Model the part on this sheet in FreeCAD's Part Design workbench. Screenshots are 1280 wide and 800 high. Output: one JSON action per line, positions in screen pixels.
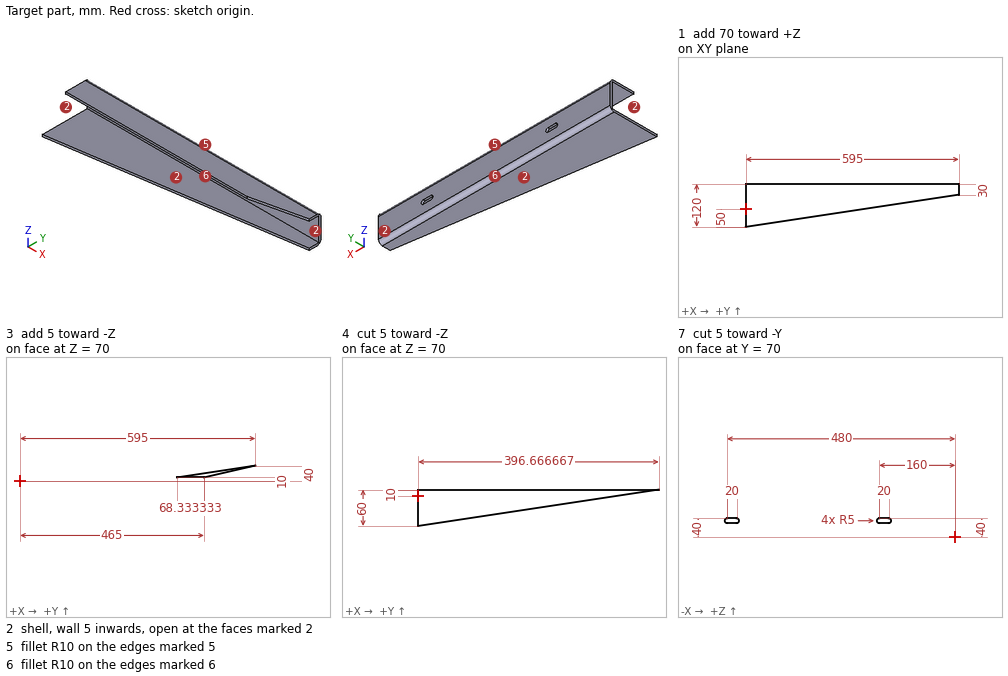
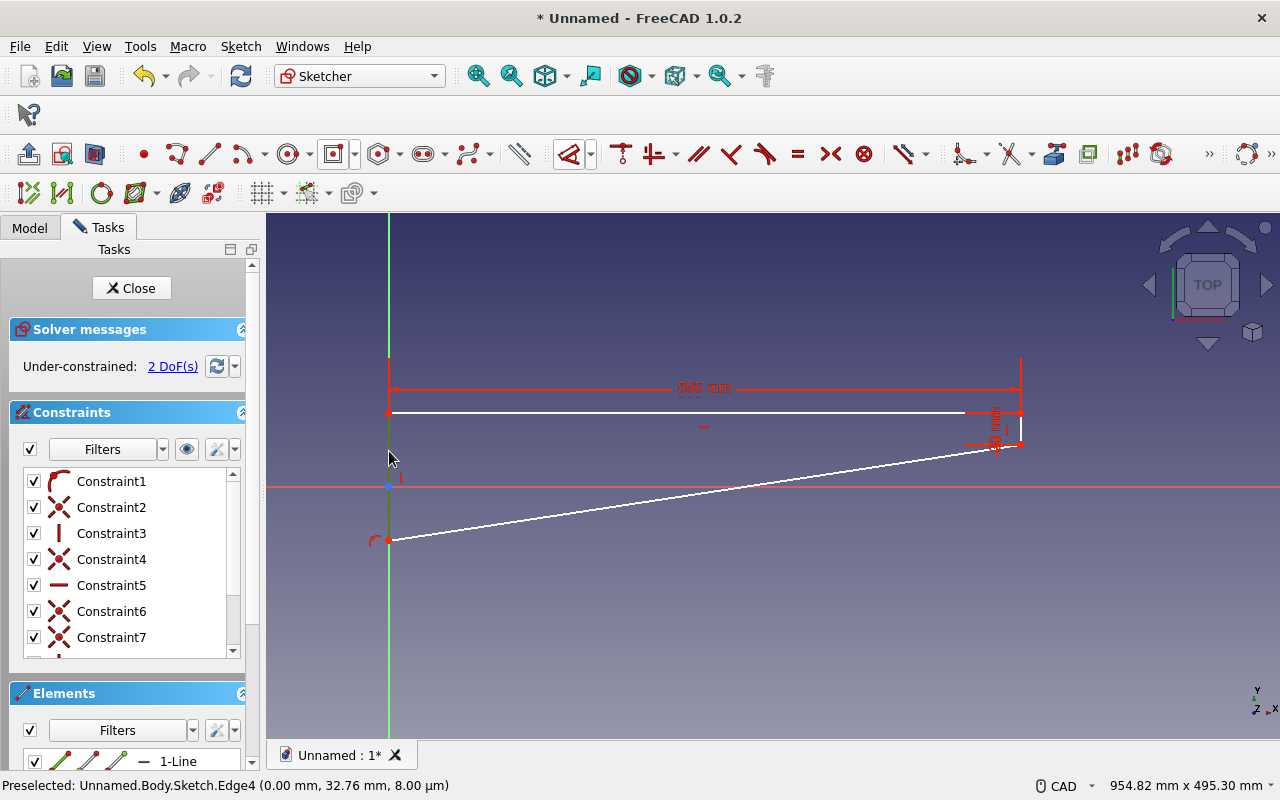
{"action": "left_click", "coordinate": [590, 154]}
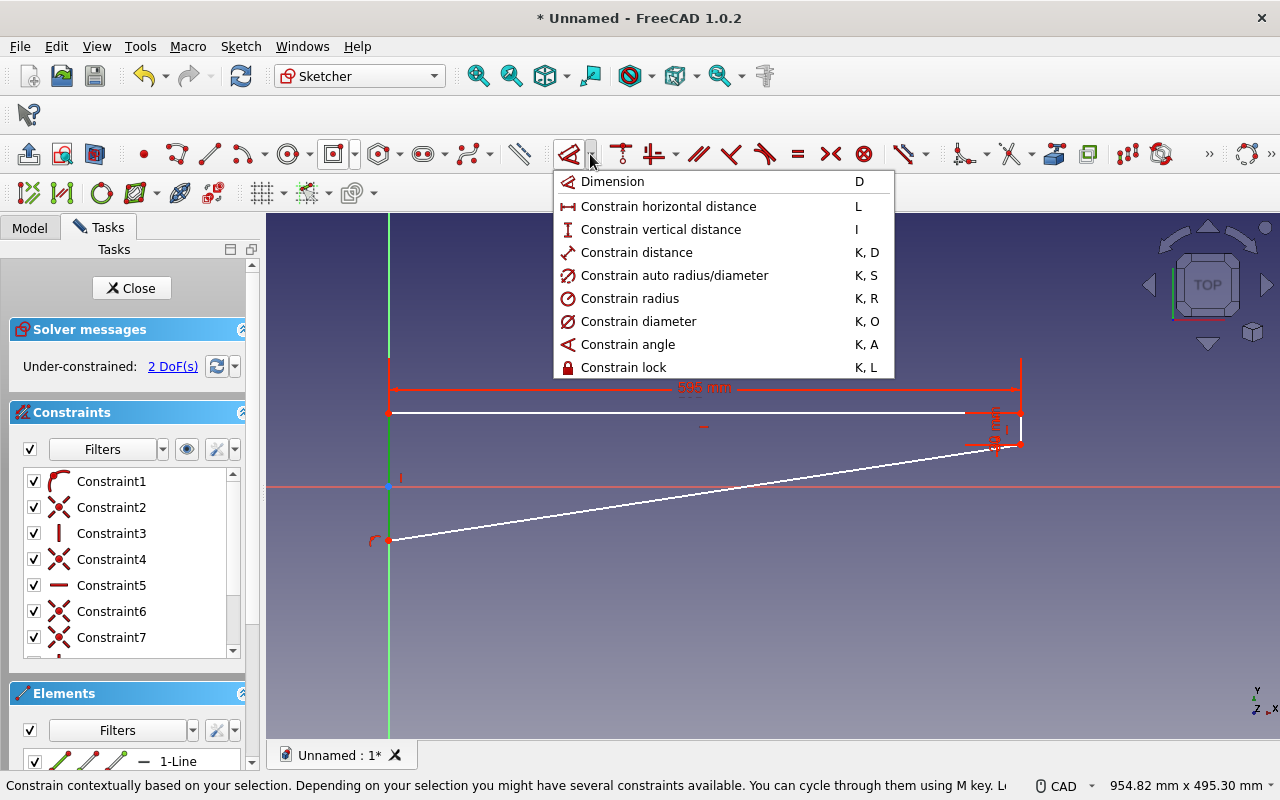
{"action": "left_click", "coordinate": [724, 230]}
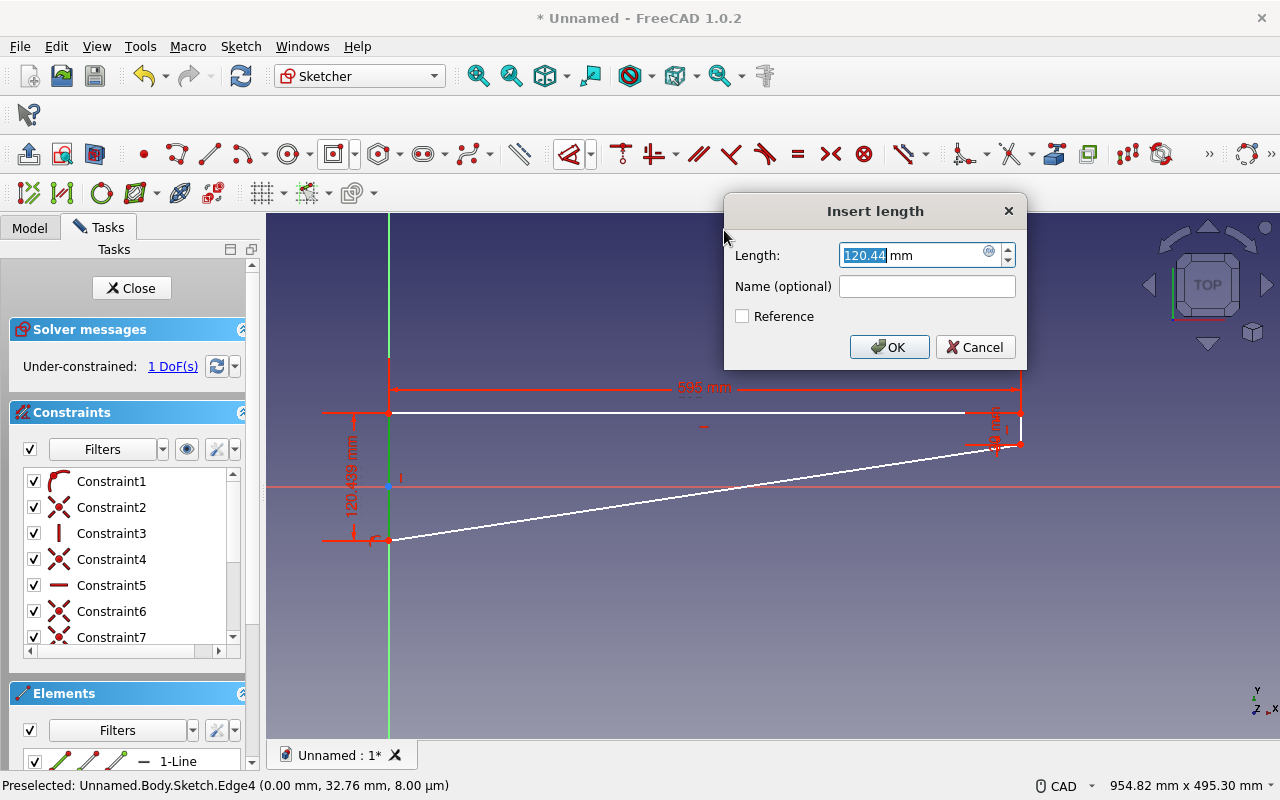
{"action": "type", "text": "120"}
{"action": "key", "text": "Return"}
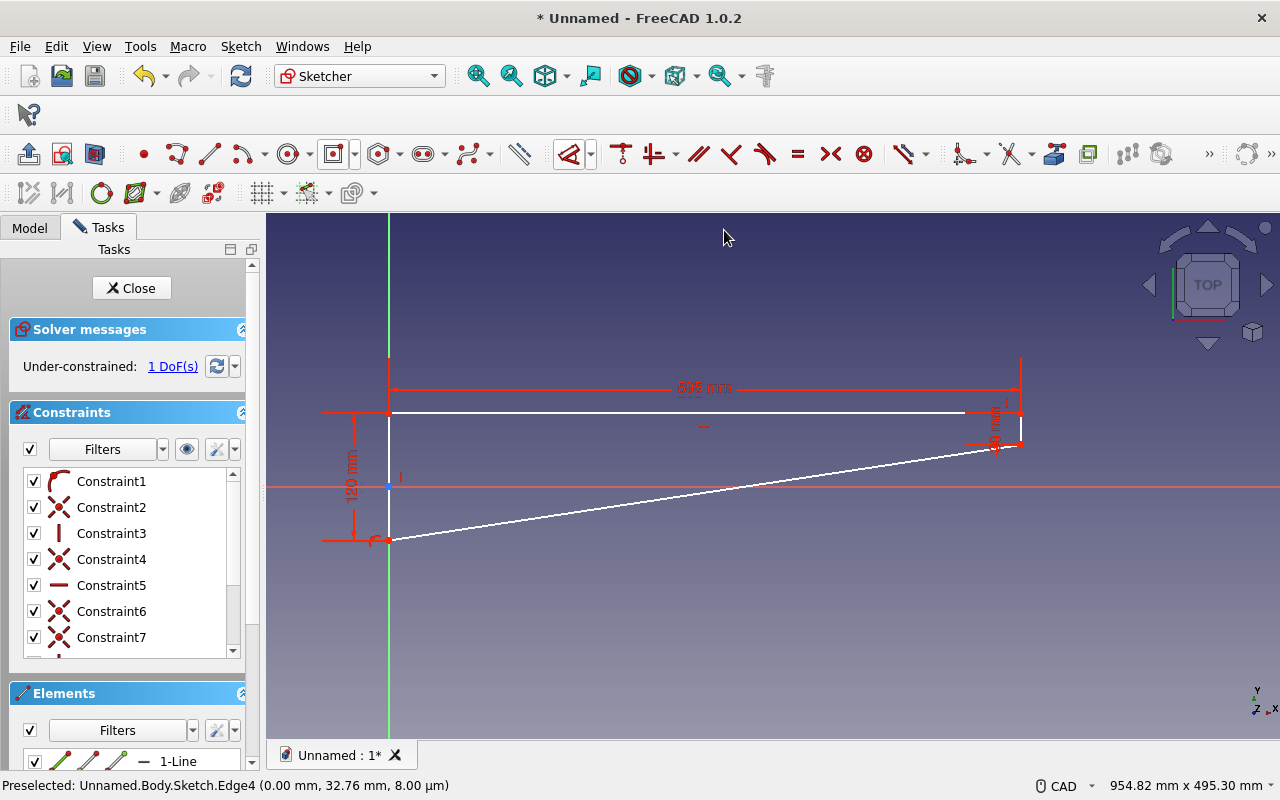
{"action": "left_click", "coordinate": [389, 541]}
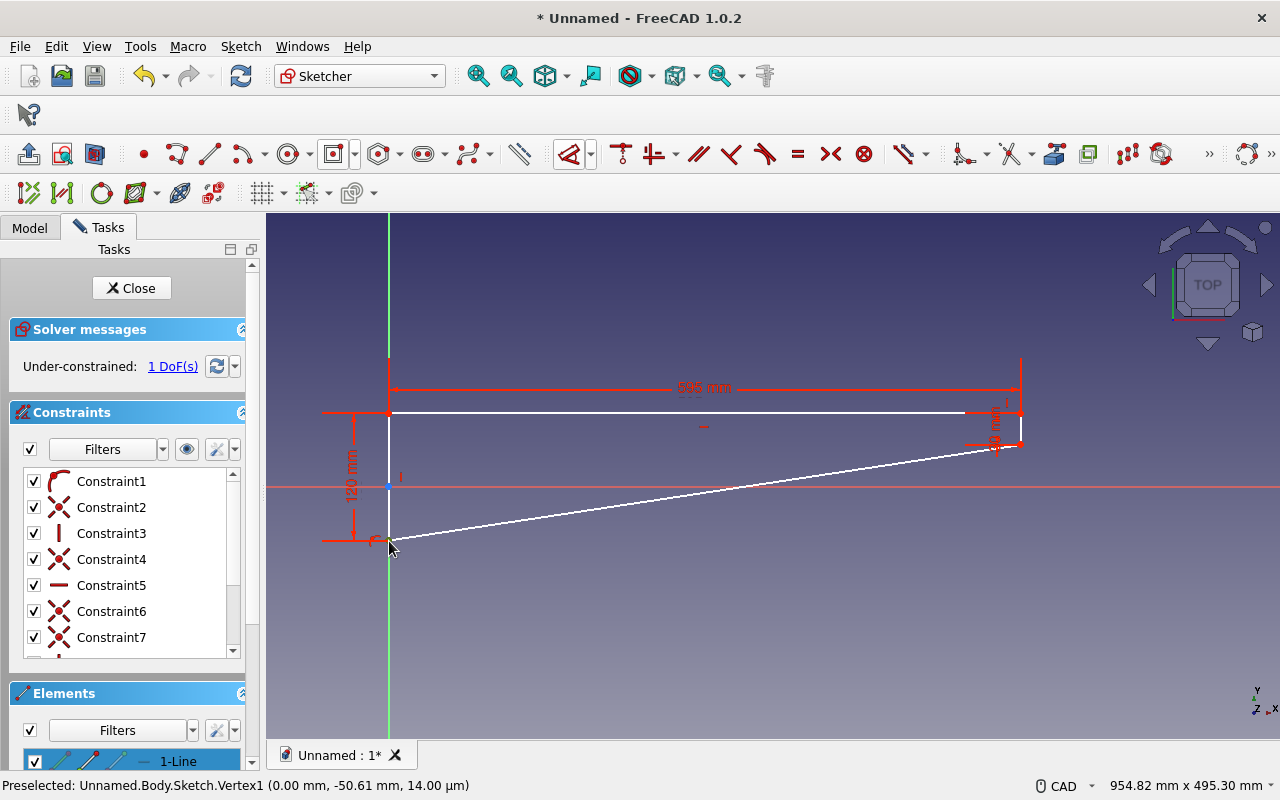
{"action": "key", "text": "i"}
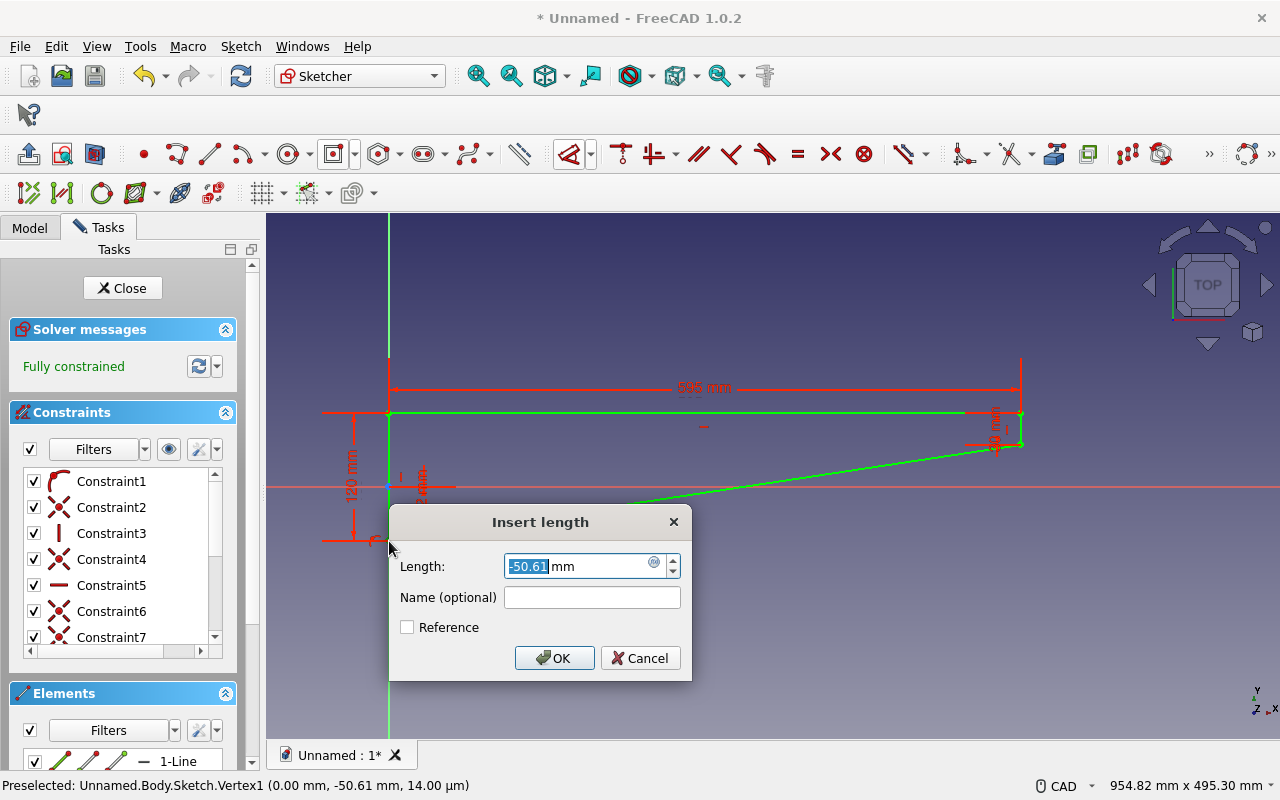
{"action": "type", "text": "-50"}
{"action": "key", "text": "Return"}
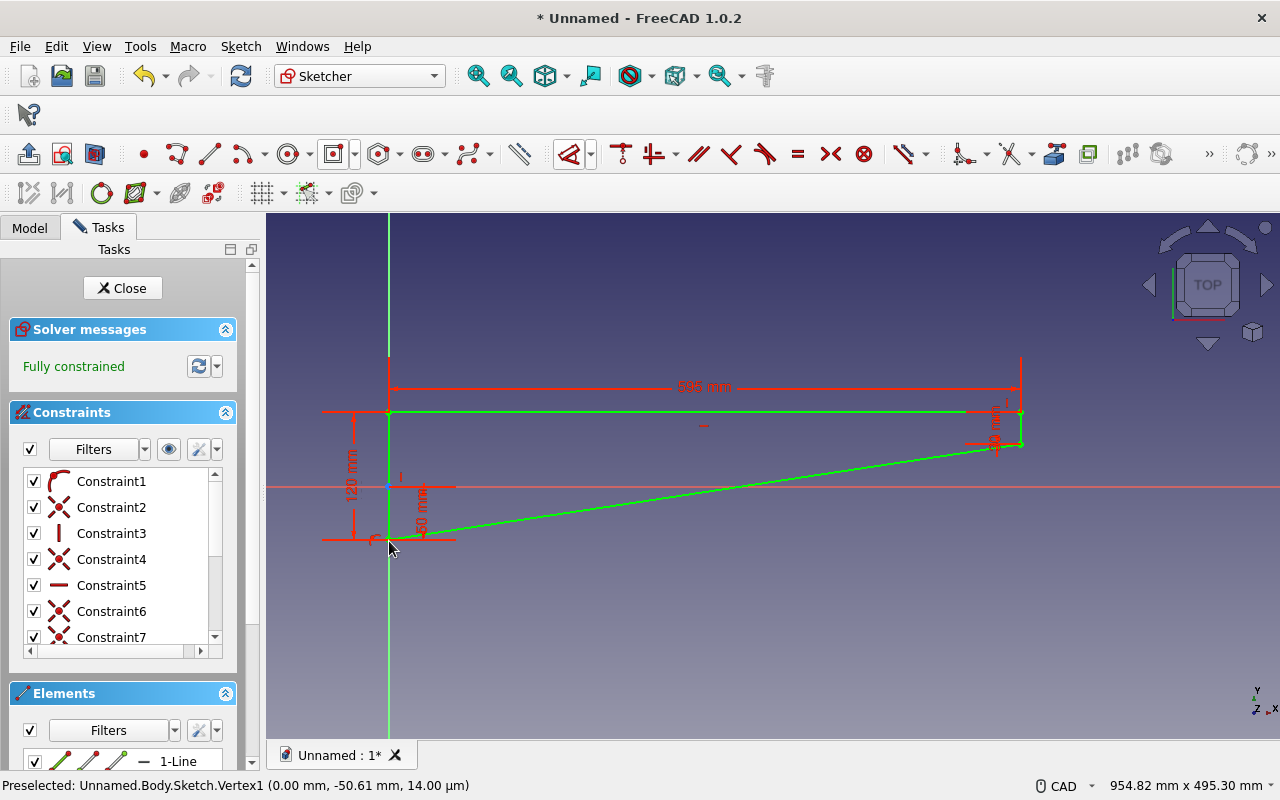
{"action": "left_click", "coordinate": [123, 288]}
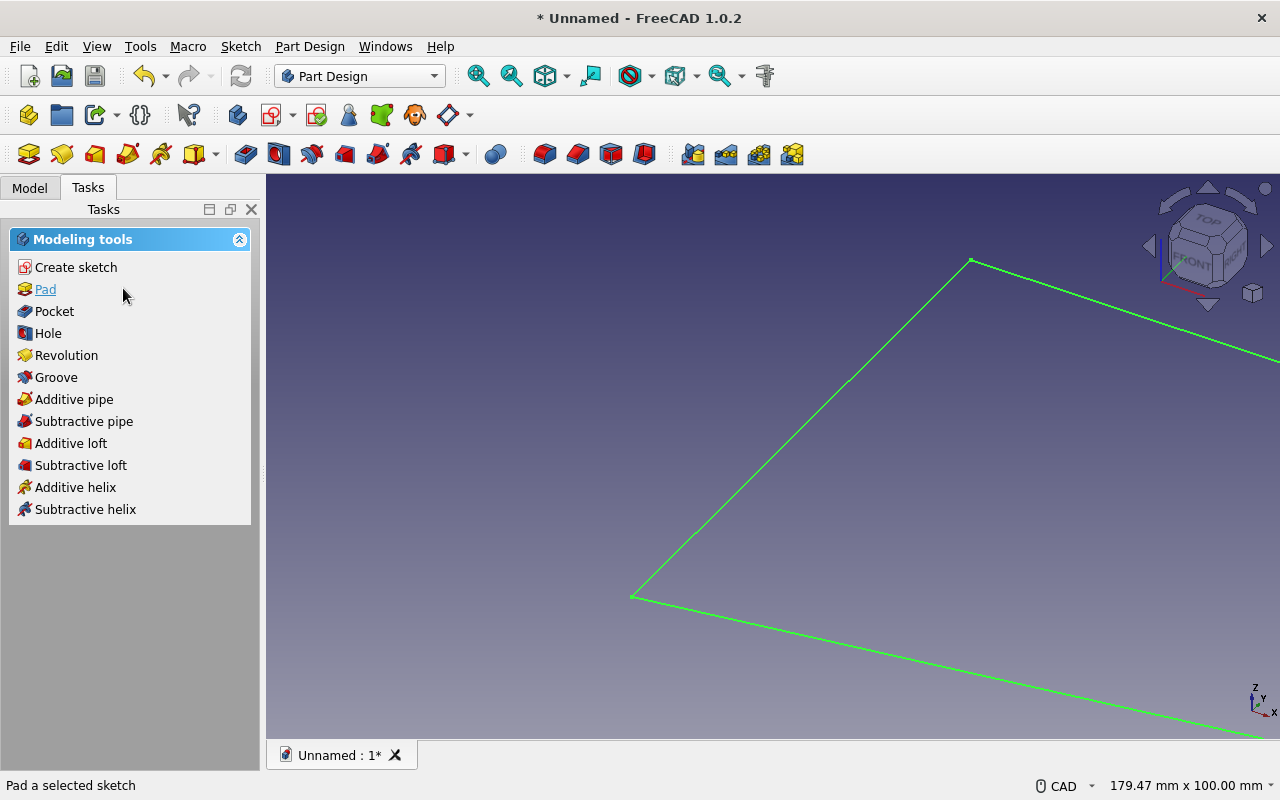
{"action": "left_click", "coordinate": [29, 154]}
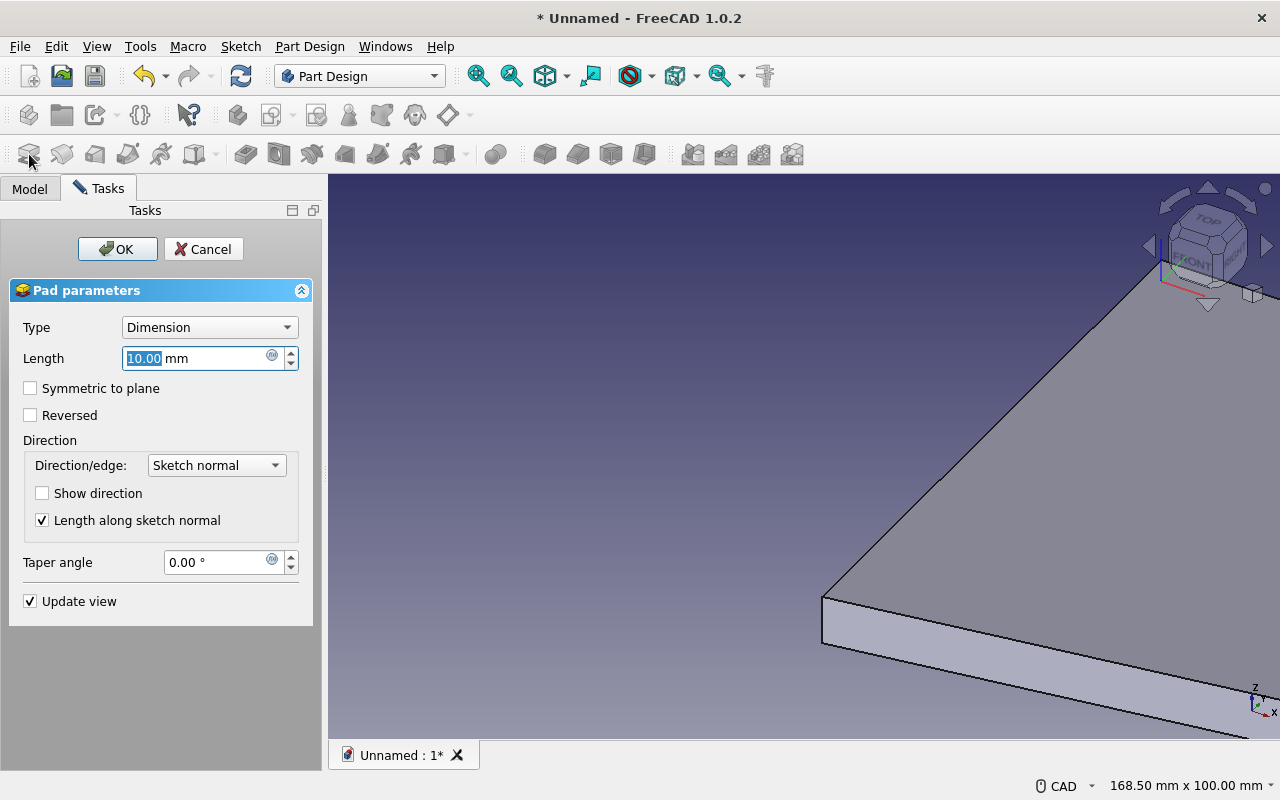
{"action": "type", "text": "70"}
{"action": "key", "text": "Tab"}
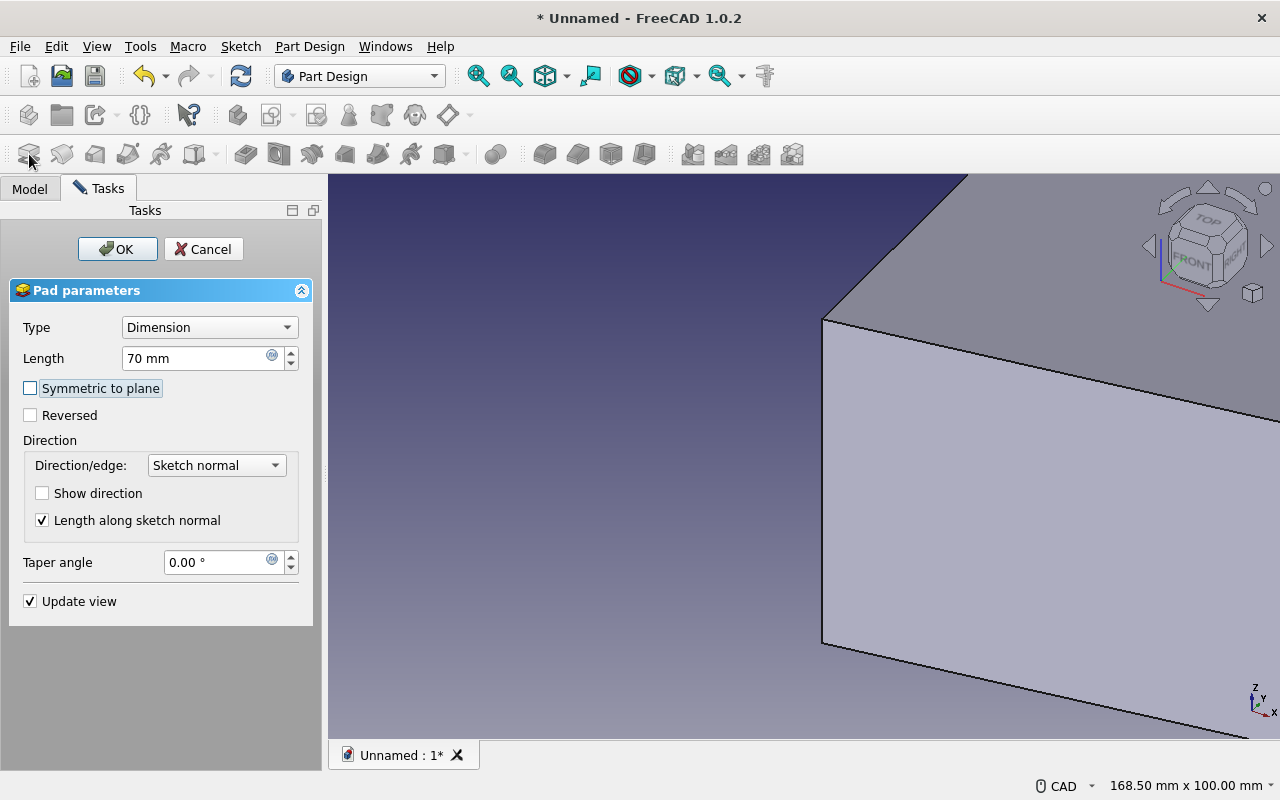
{"action": "left_click", "coordinate": [118, 249]}